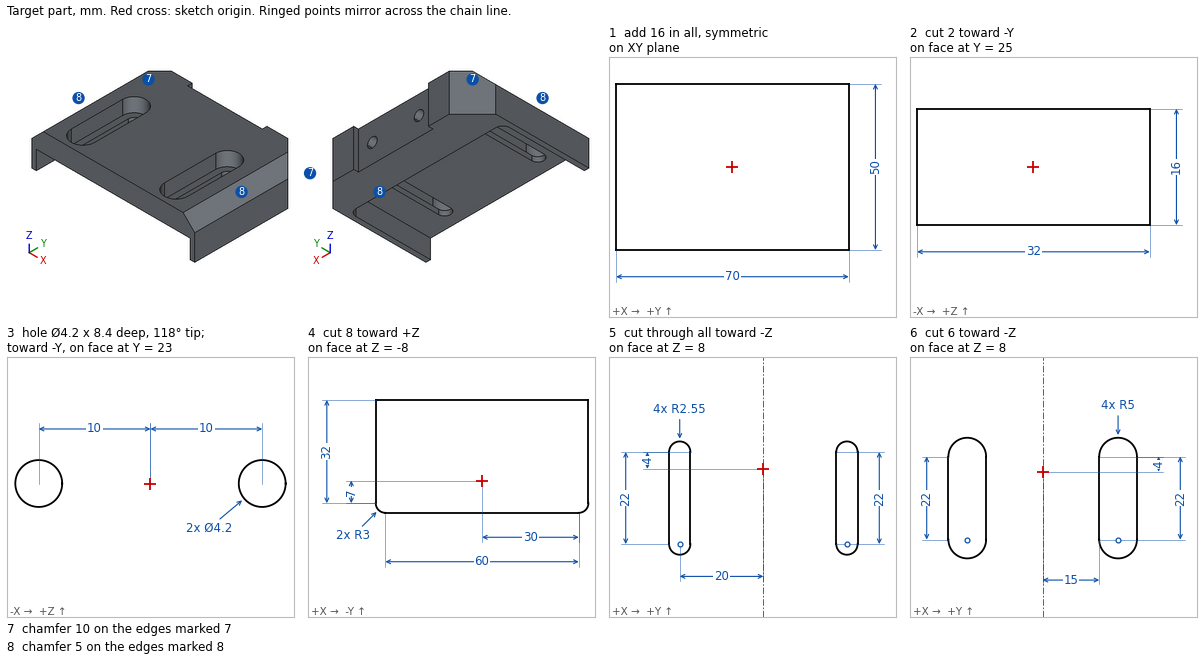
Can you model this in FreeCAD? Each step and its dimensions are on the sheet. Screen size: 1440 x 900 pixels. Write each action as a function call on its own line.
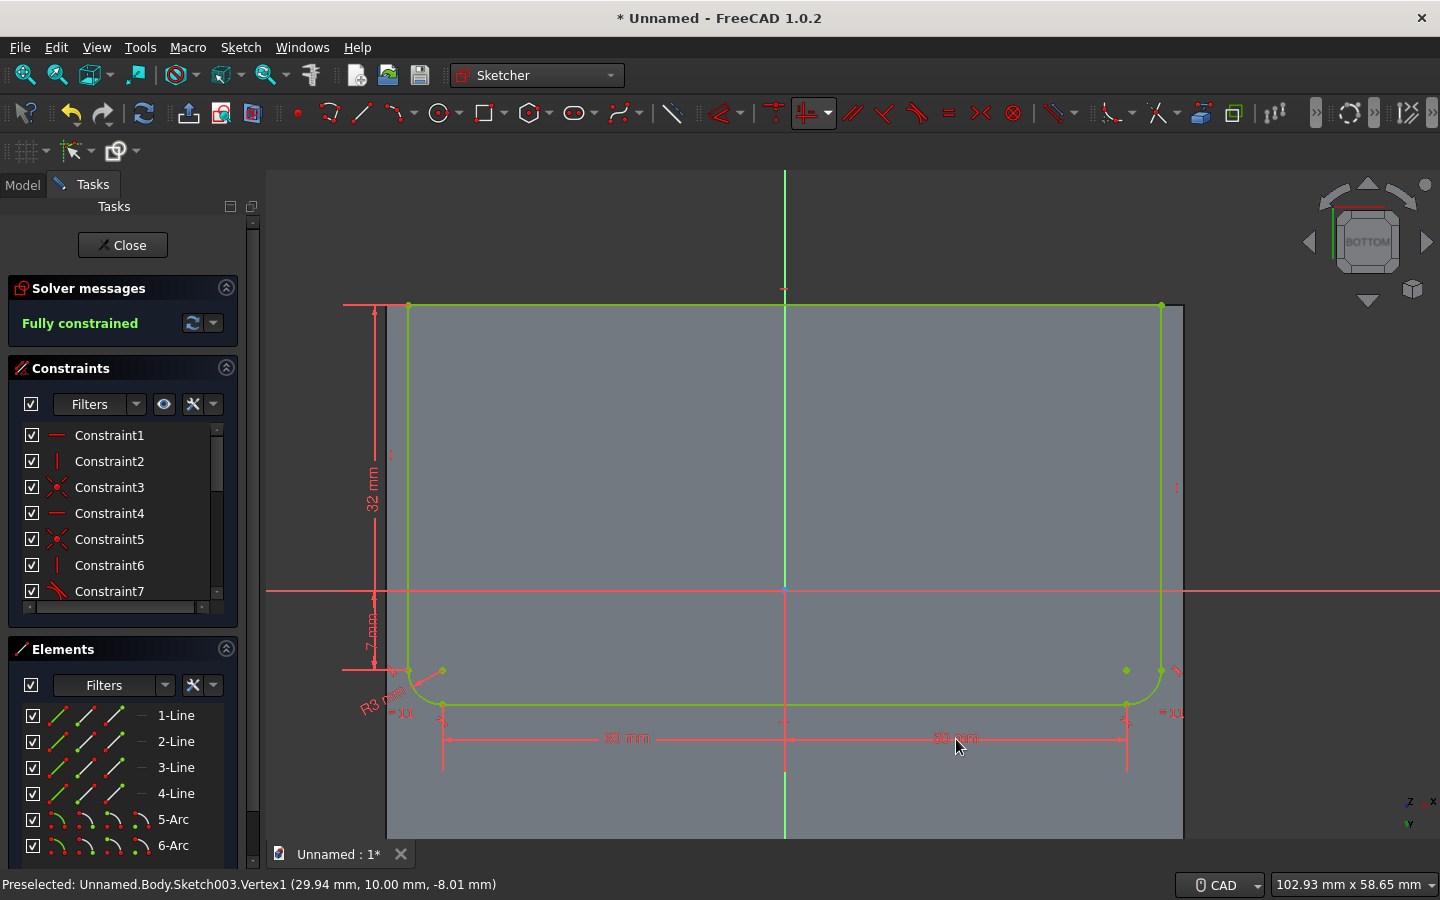
click(123, 245)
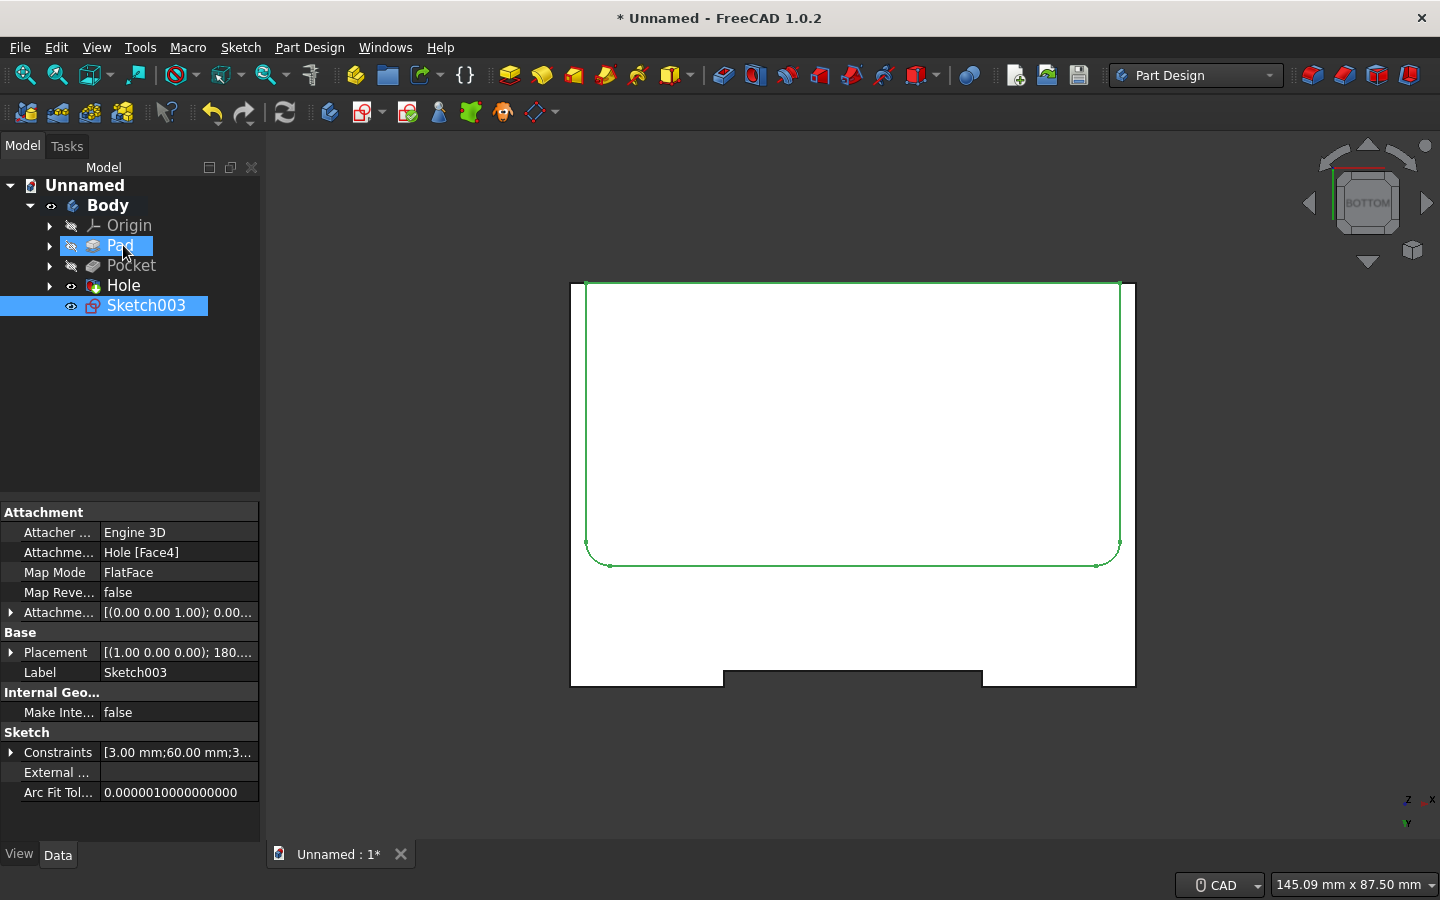
click(724, 76)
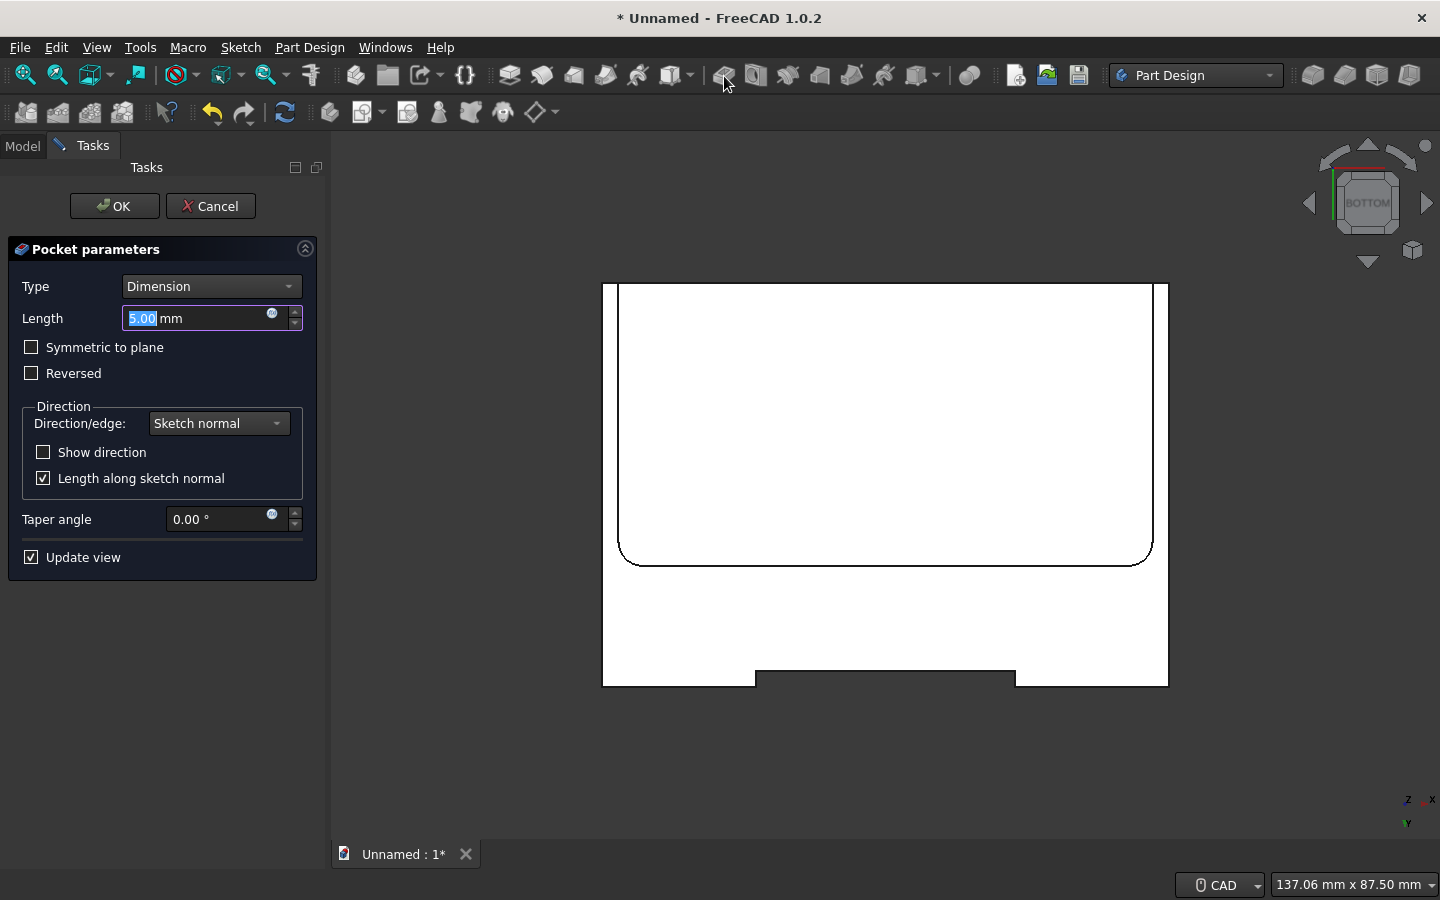
text(8)
key(Tab)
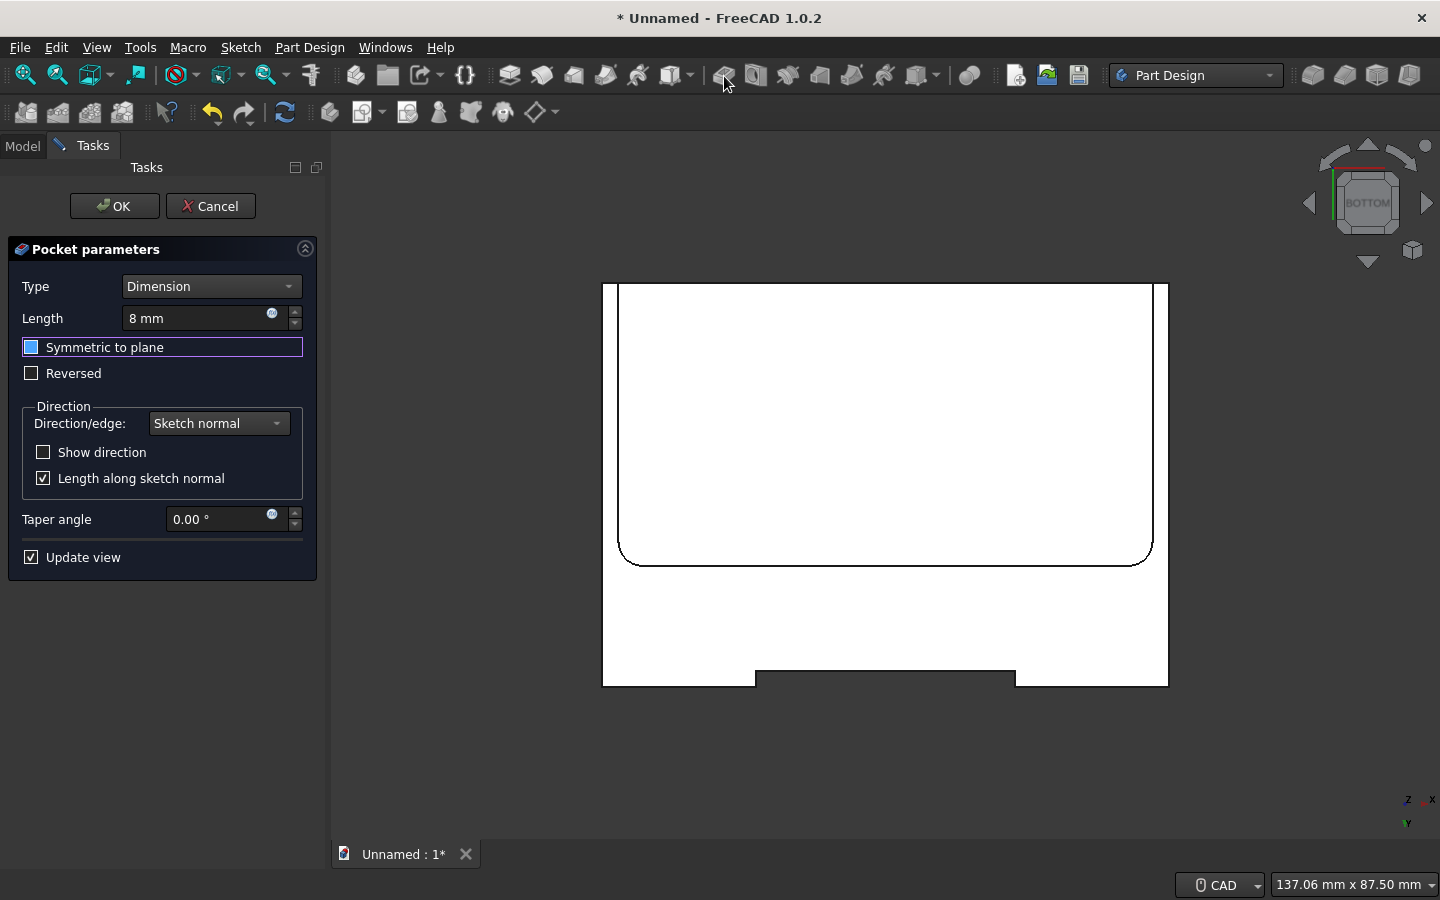
click(115, 206)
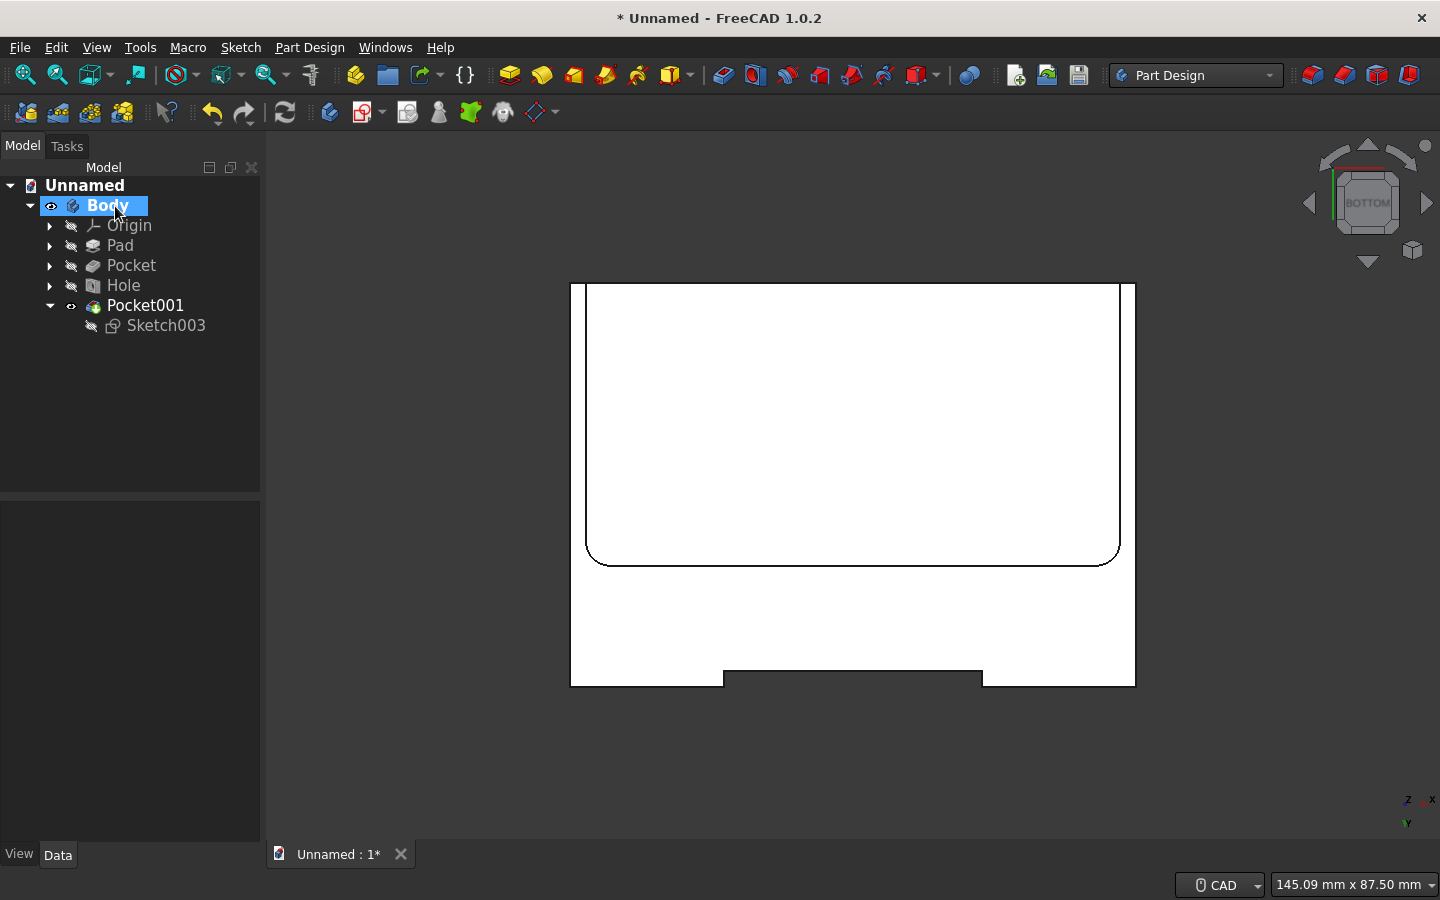
key(0)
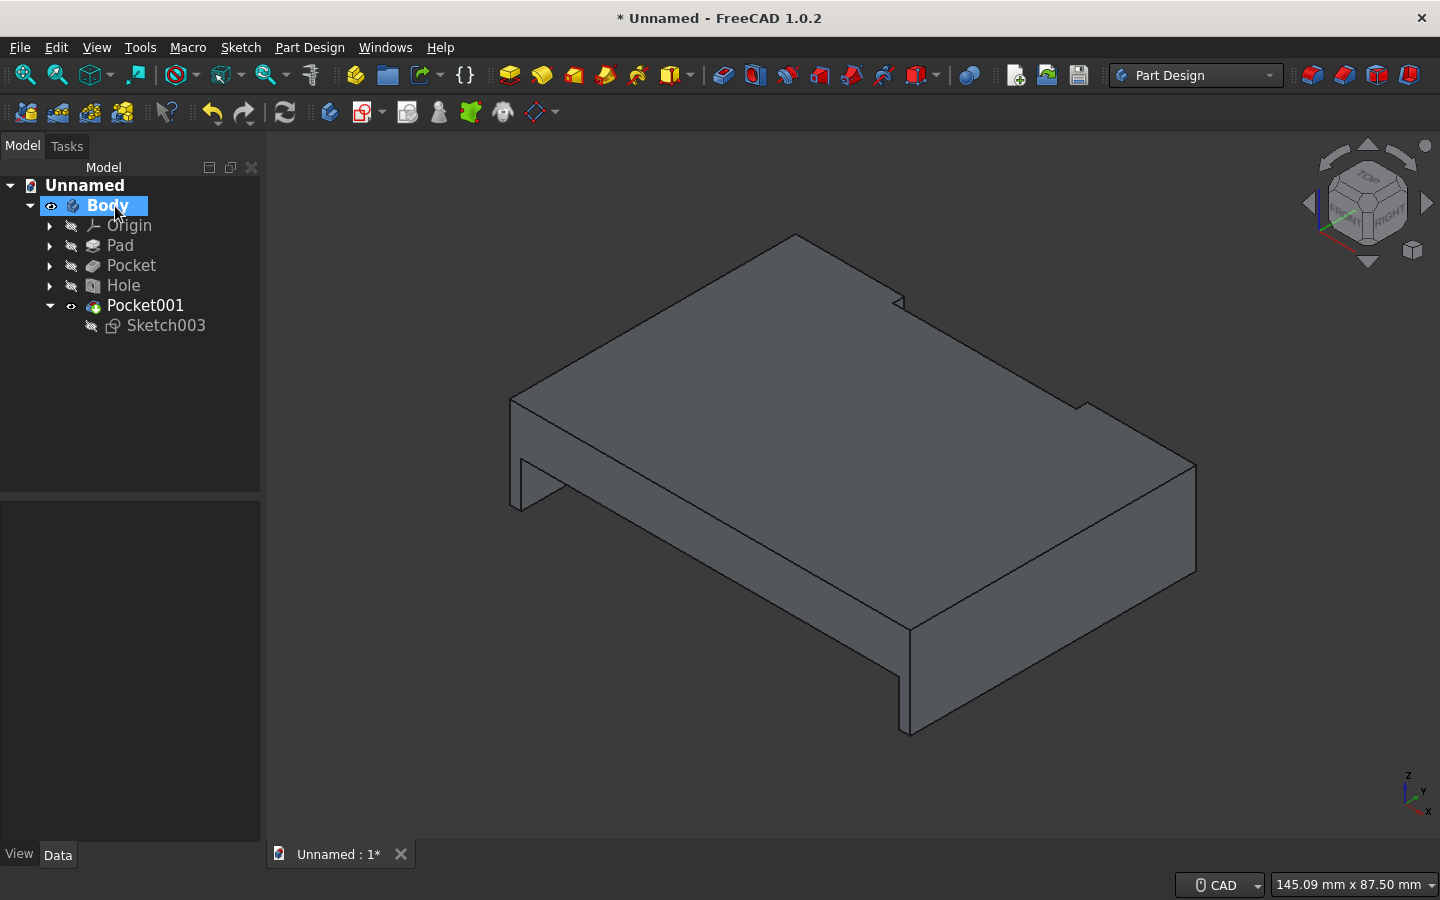
click(910, 464)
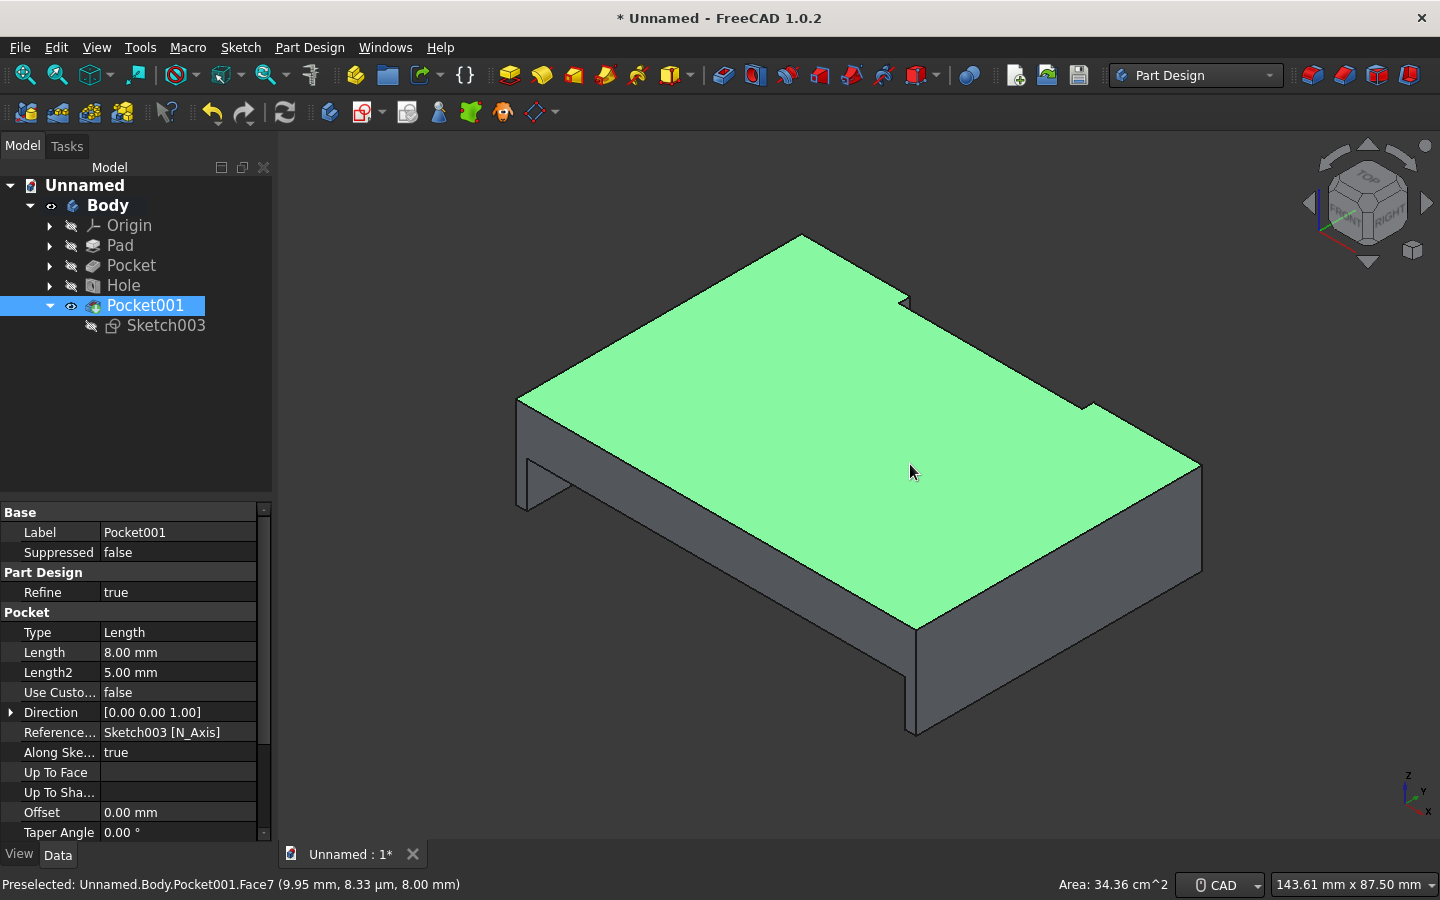
click(362, 112)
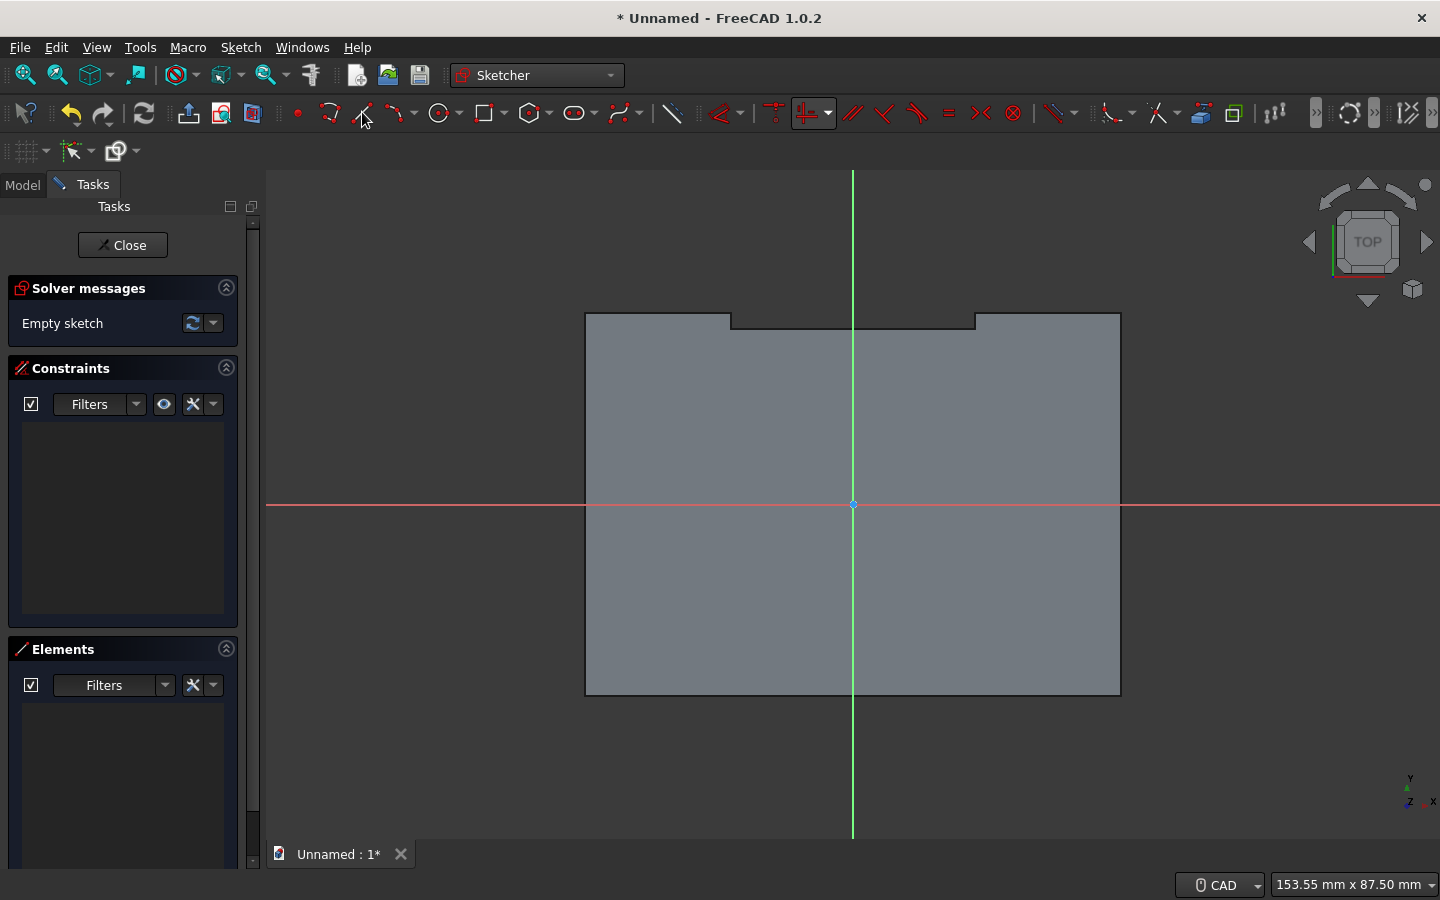
scroll(936, 623, up, 3)